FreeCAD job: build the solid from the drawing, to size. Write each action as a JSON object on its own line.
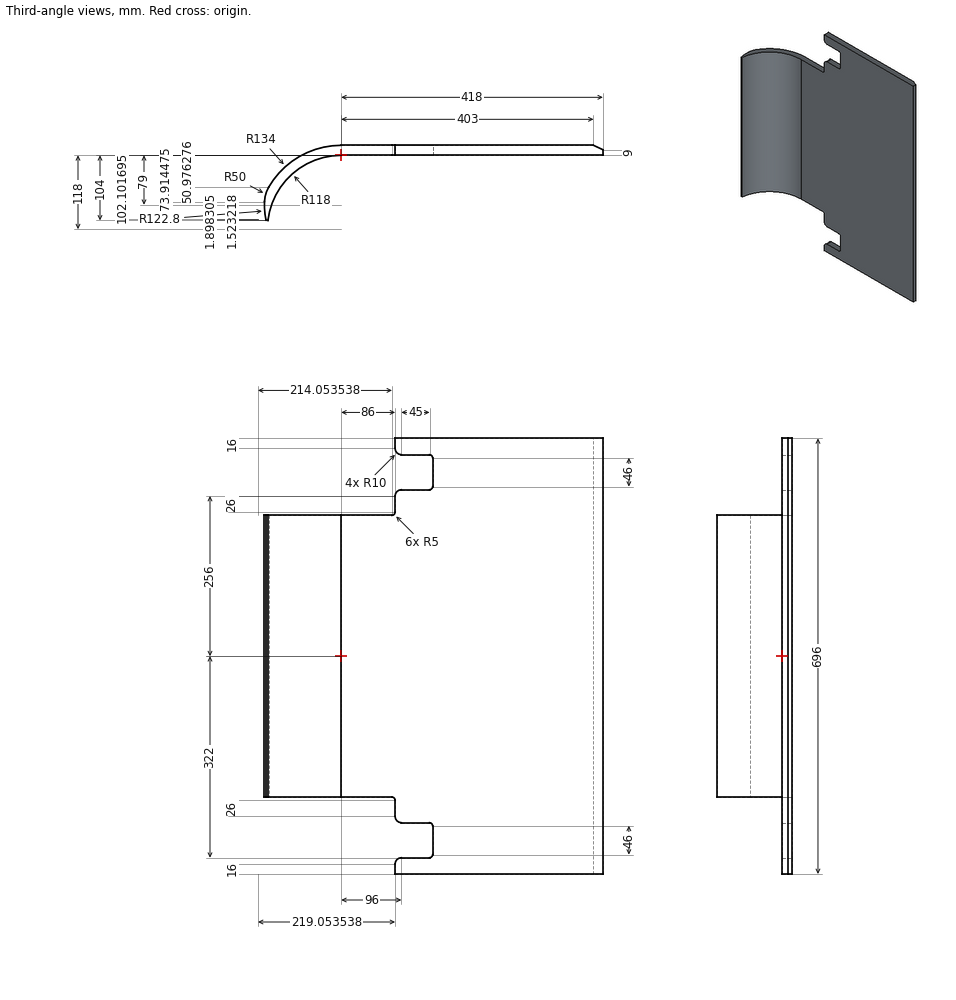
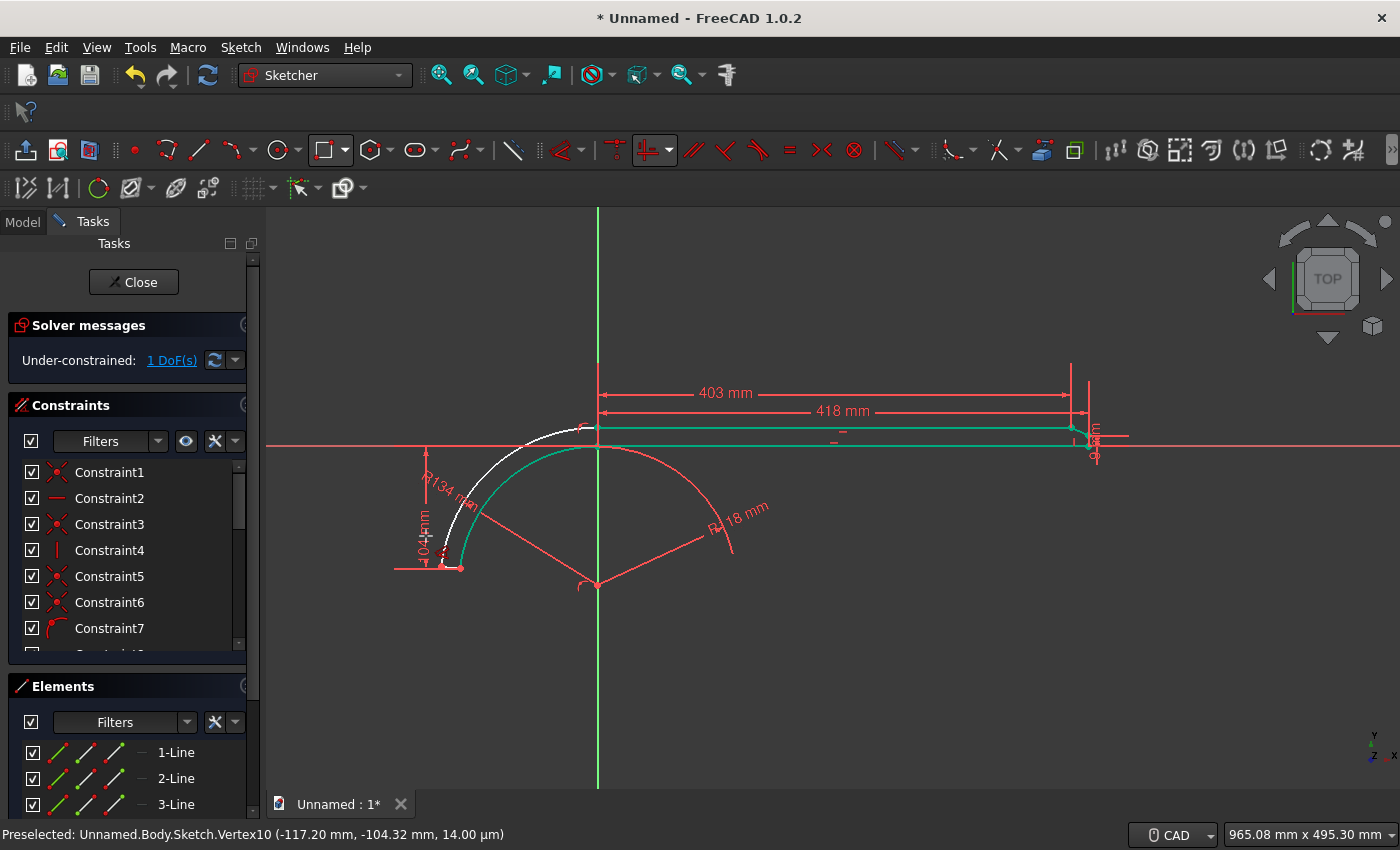
{"action": "scroll", "coordinate": [451, 568], "scroll_direction": "up", "scroll_amount": 15}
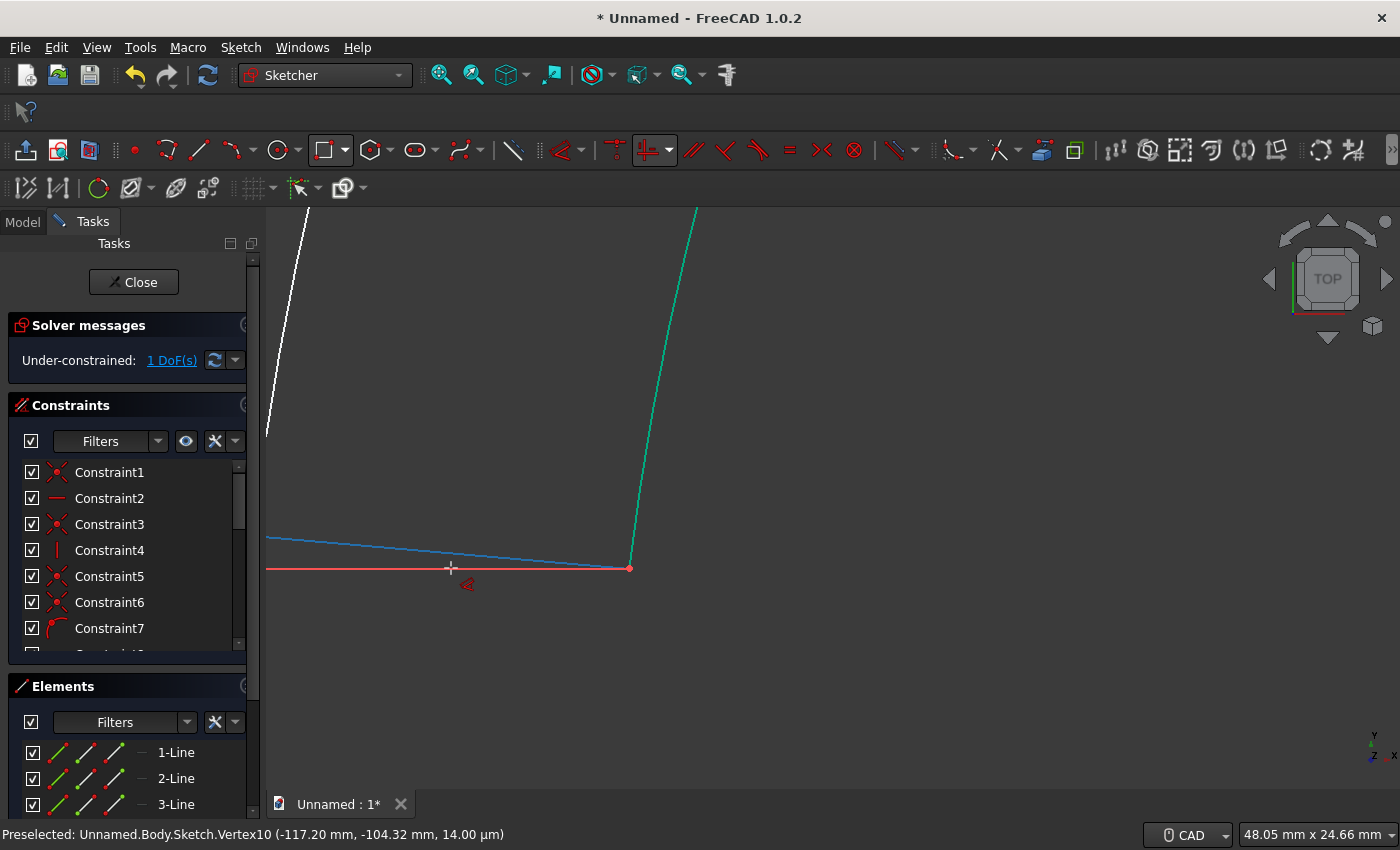
{"action": "left_click", "coordinate": [441, 553]}
{"action": "left_click", "coordinate": [663, 553]}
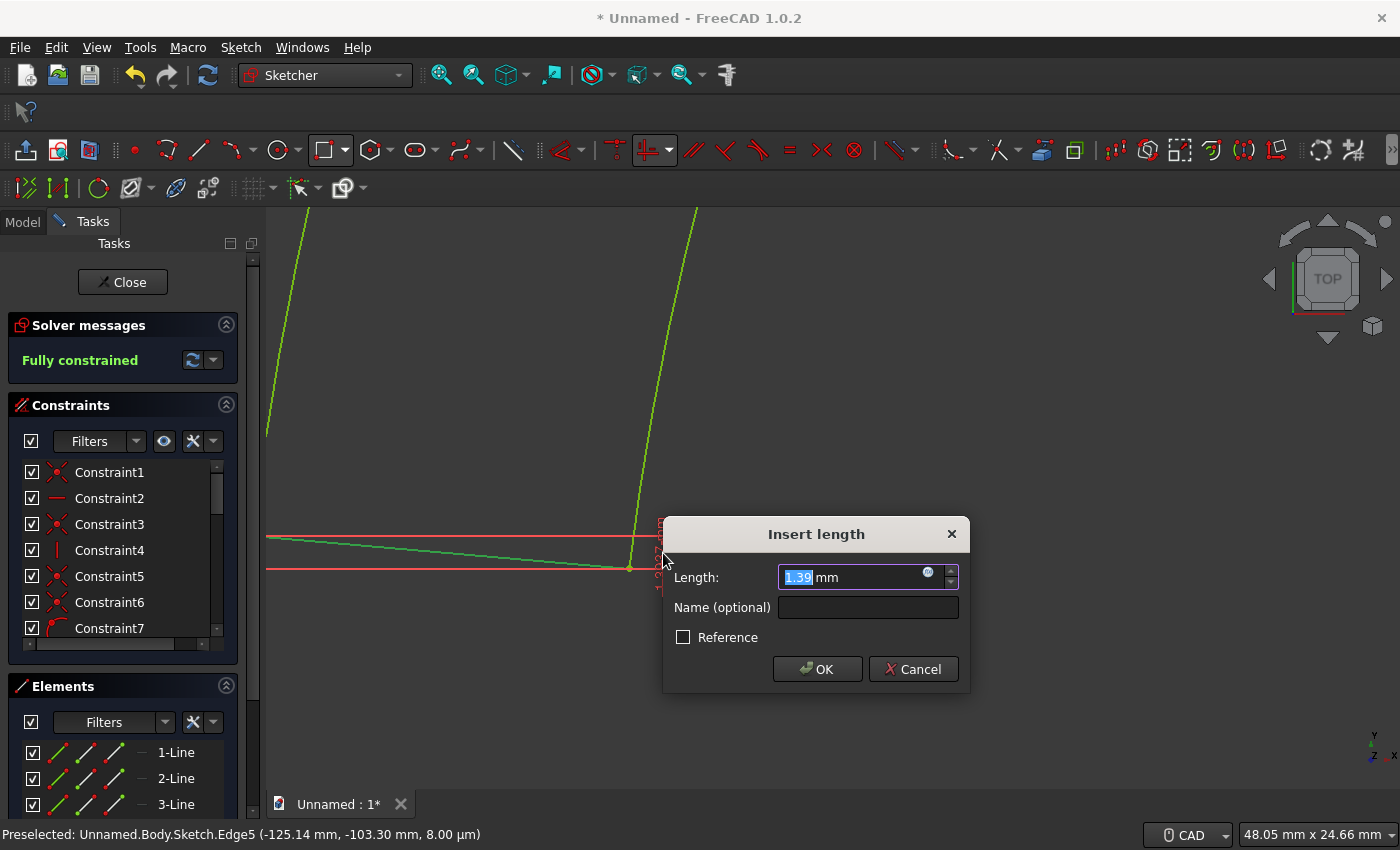
{"action": "type", "text": "1.898305"}
{"action": "key", "text": "Return"}
{"action": "key", "text": "Escape"}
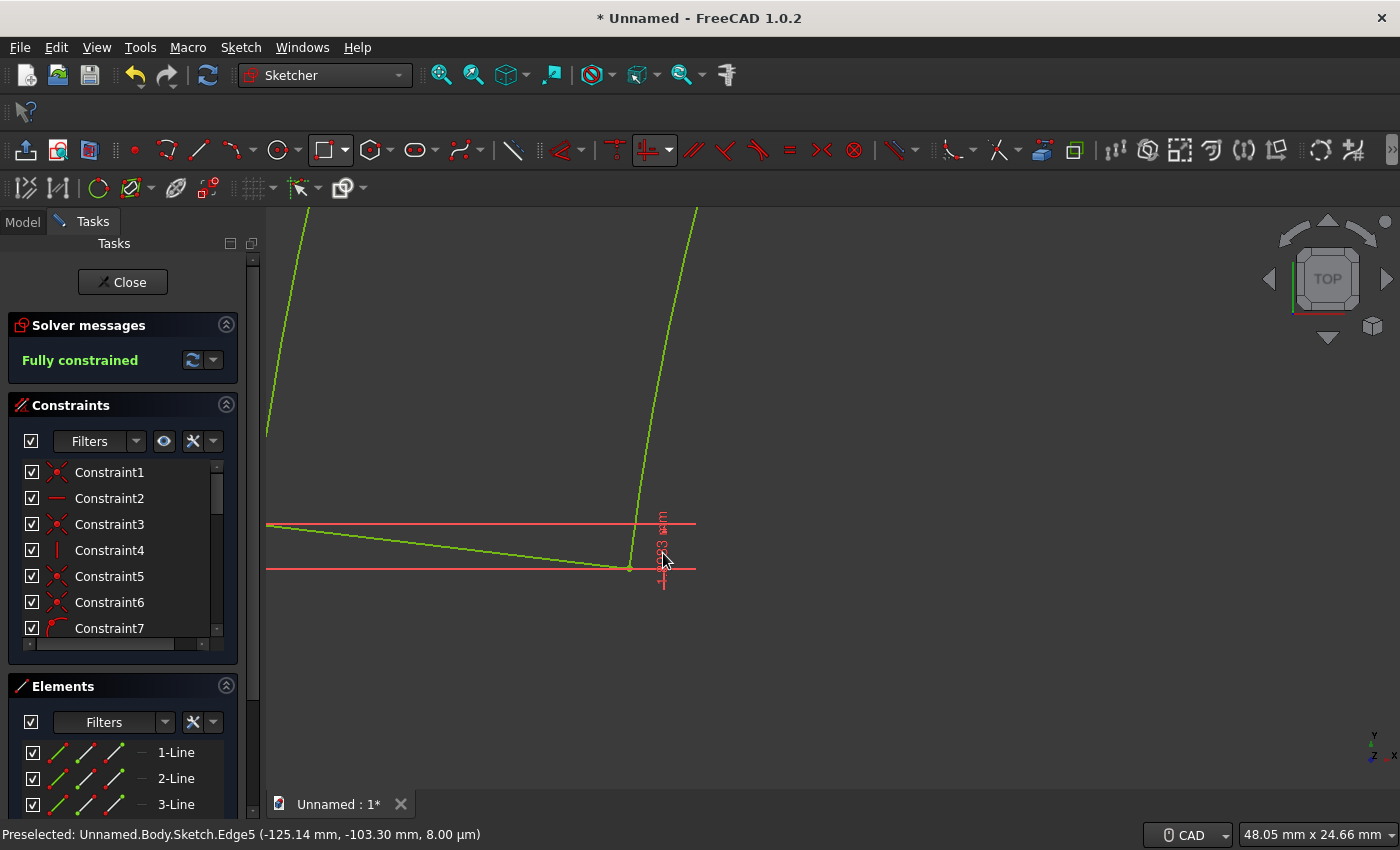
{"action": "left_click", "coordinate": [123, 282]}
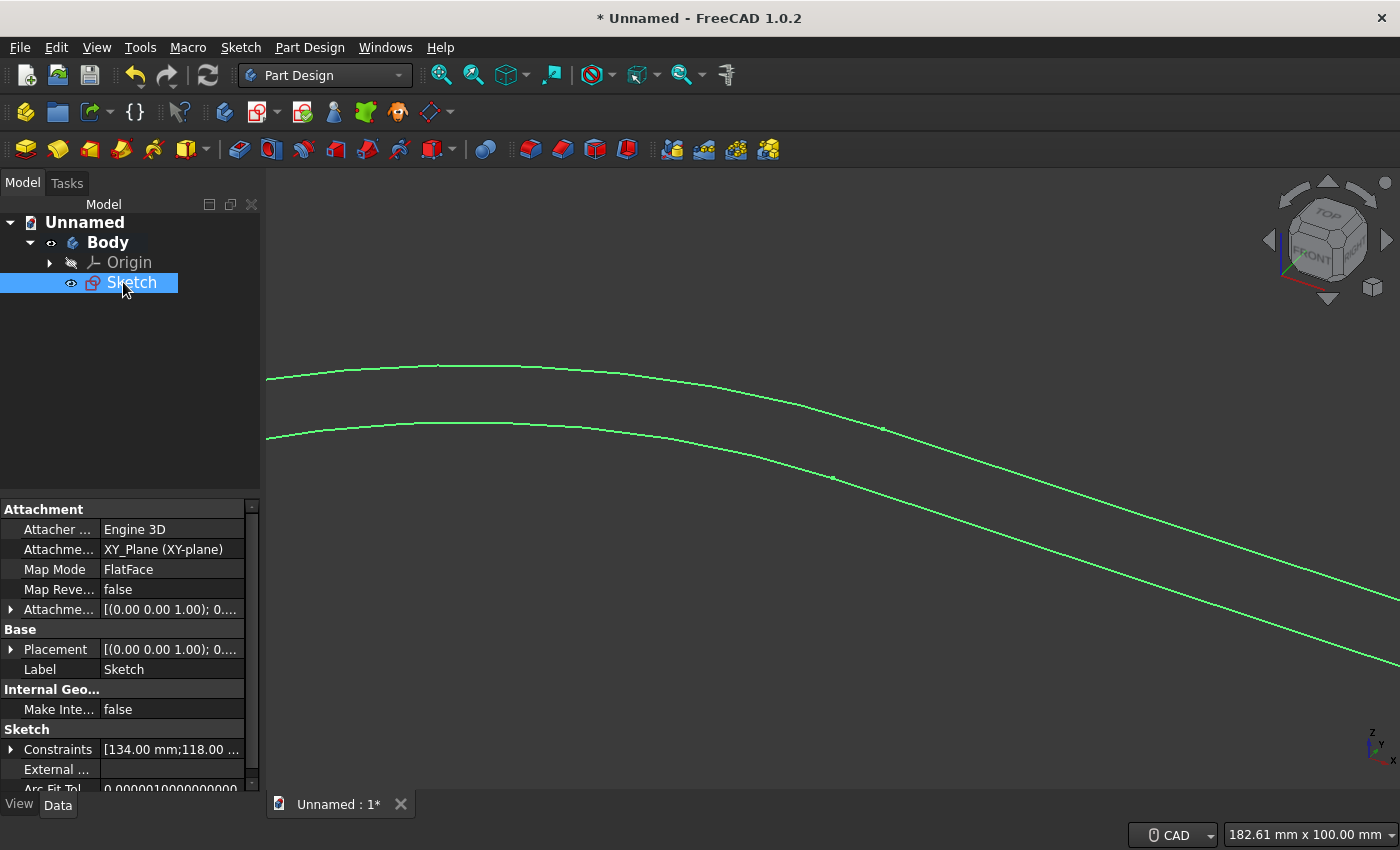
{"action": "left_click", "coordinate": [26, 150]}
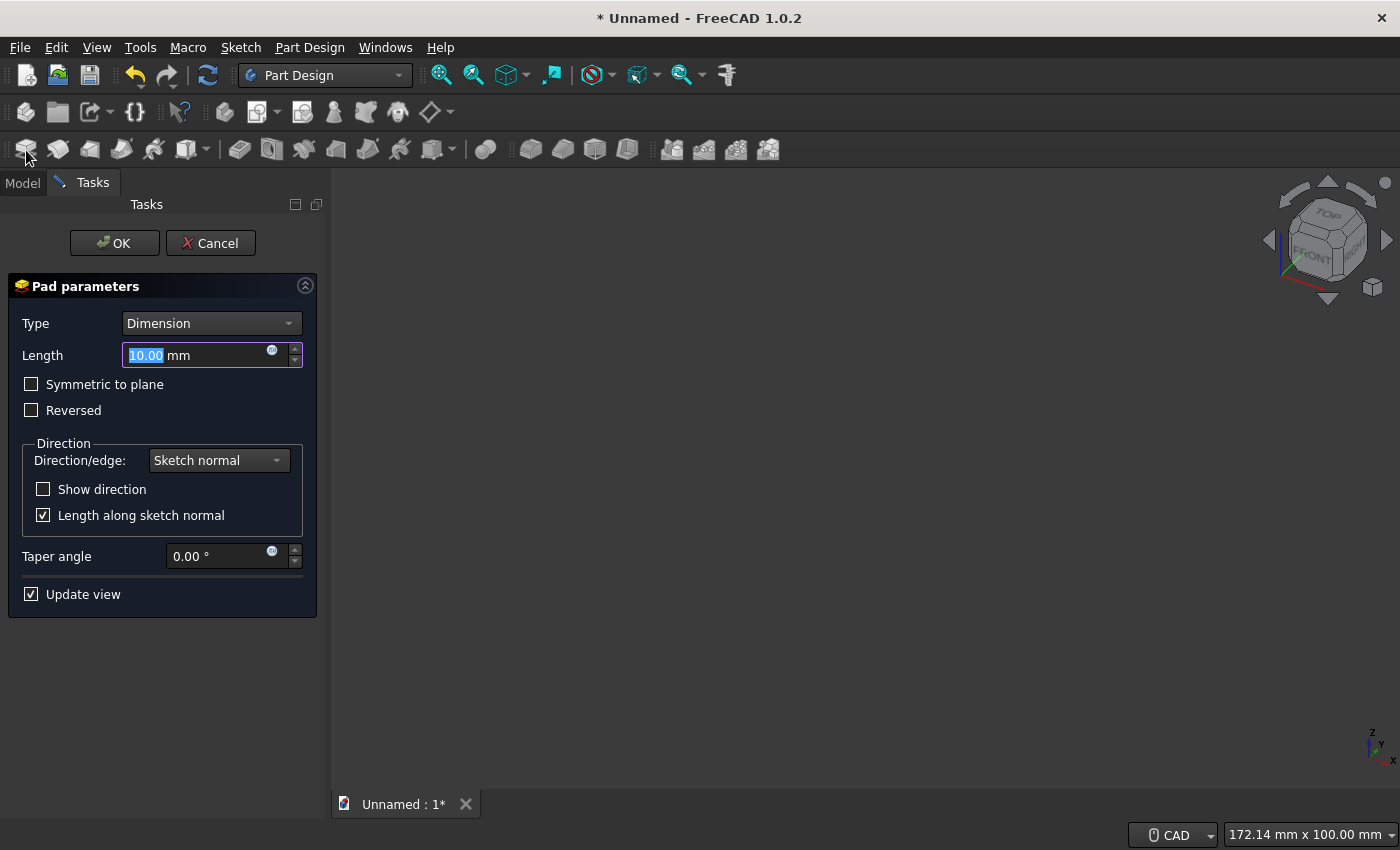
{"action": "type", "text": "696"}
{"action": "key", "text": "Tab"}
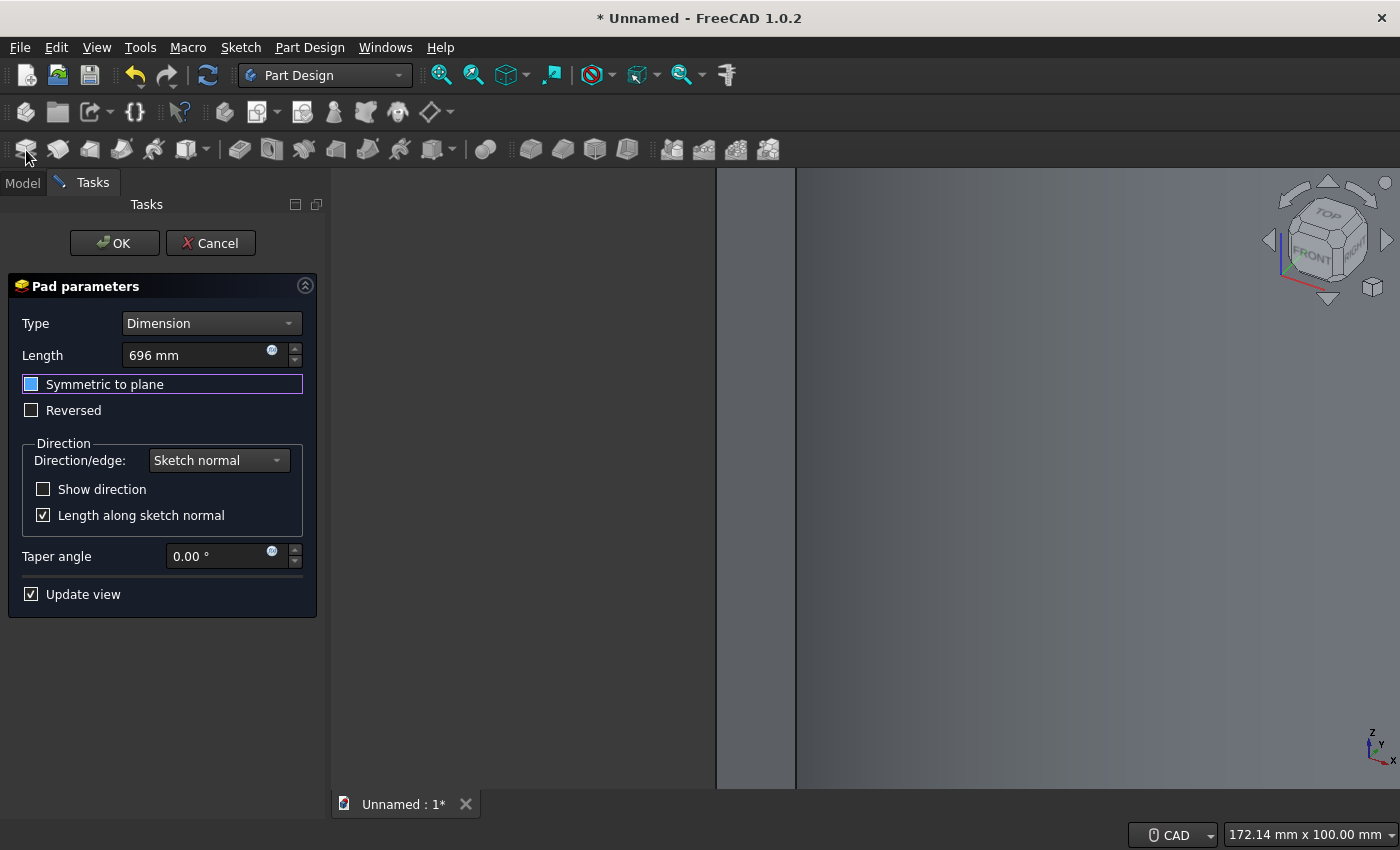
{"action": "left_click", "coordinate": [30, 384]}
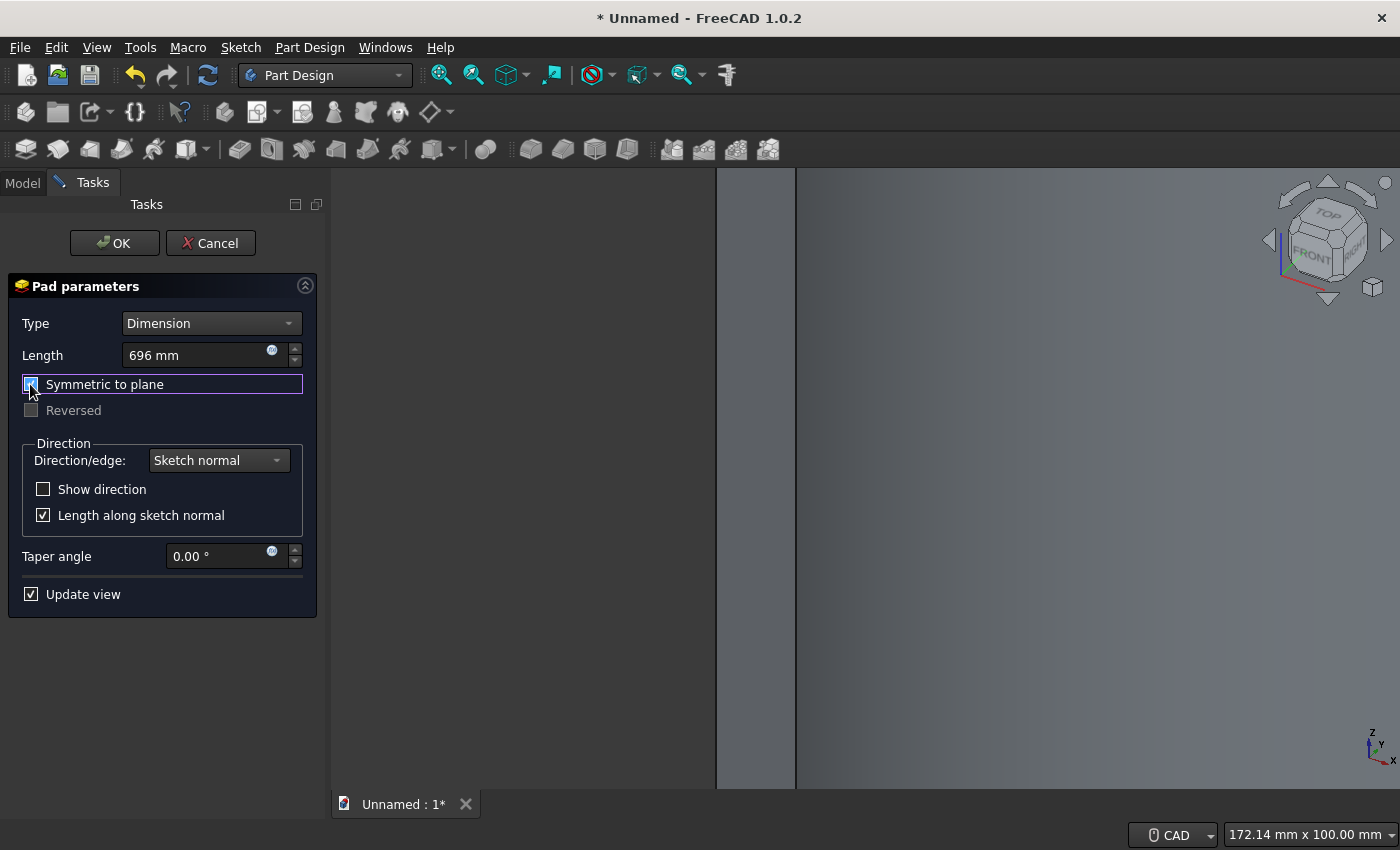
{"action": "left_click", "coordinate": [115, 243]}